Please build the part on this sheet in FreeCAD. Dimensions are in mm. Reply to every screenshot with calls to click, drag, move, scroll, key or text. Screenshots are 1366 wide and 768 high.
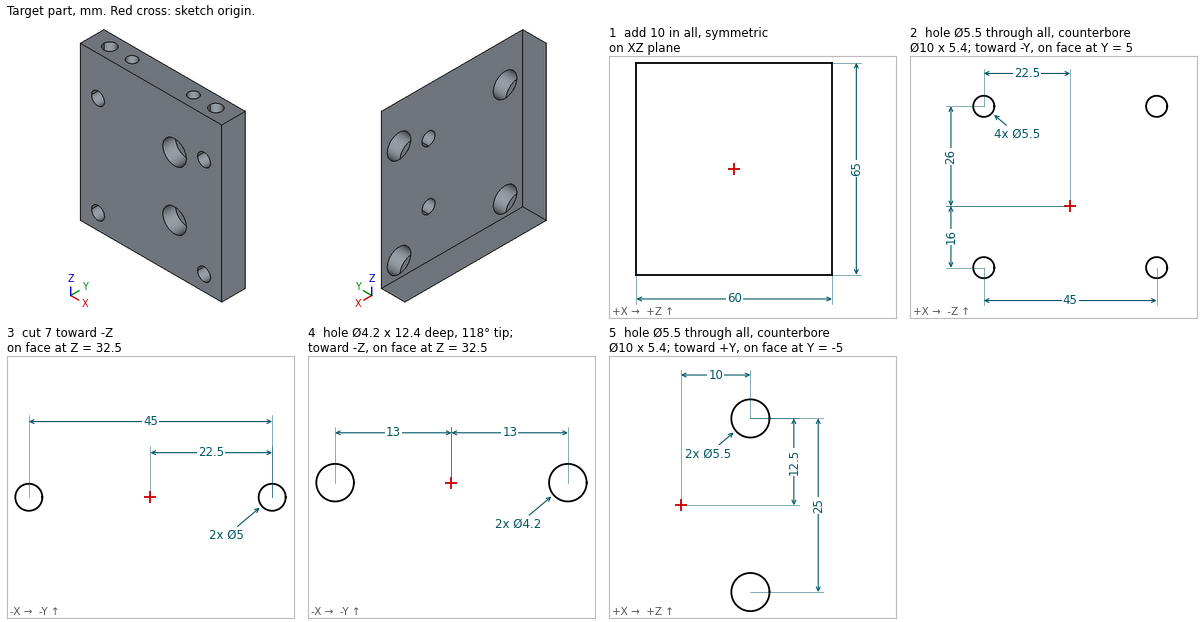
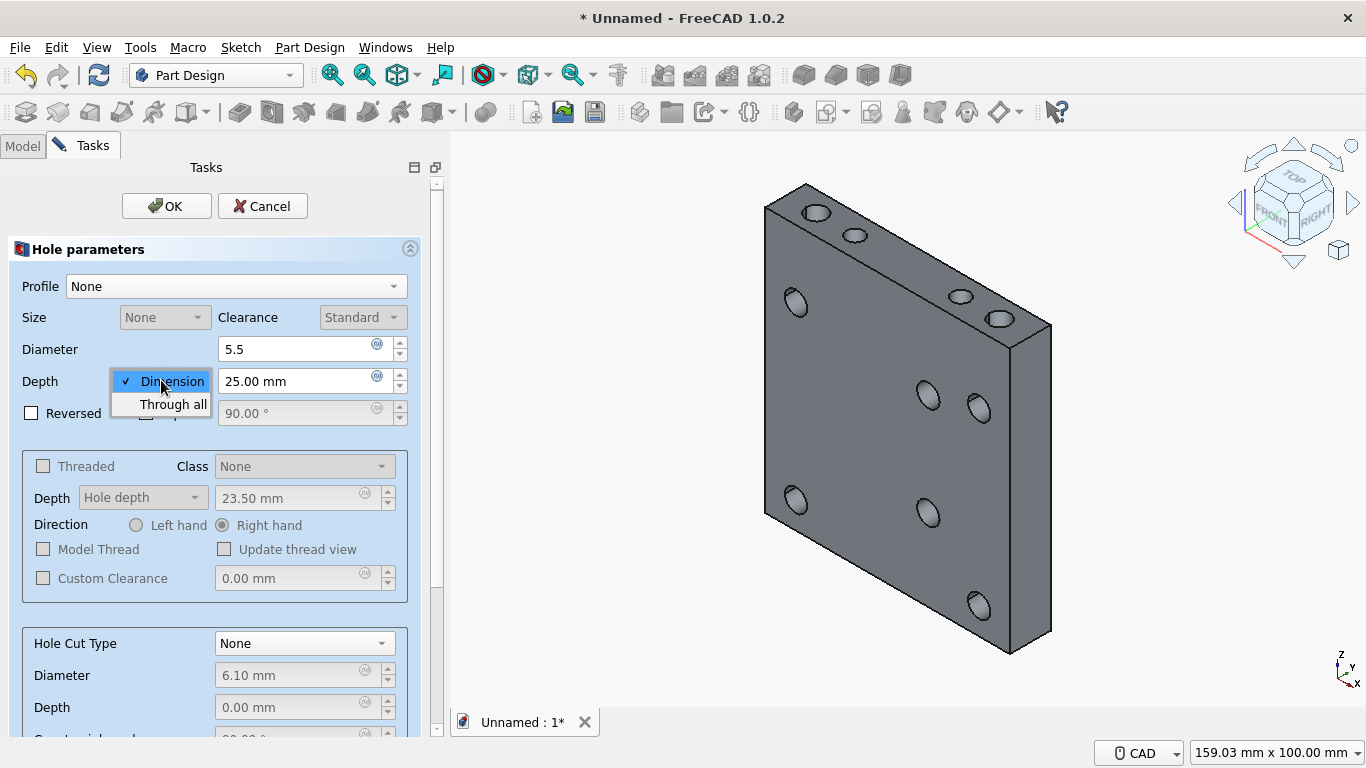
click(160, 404)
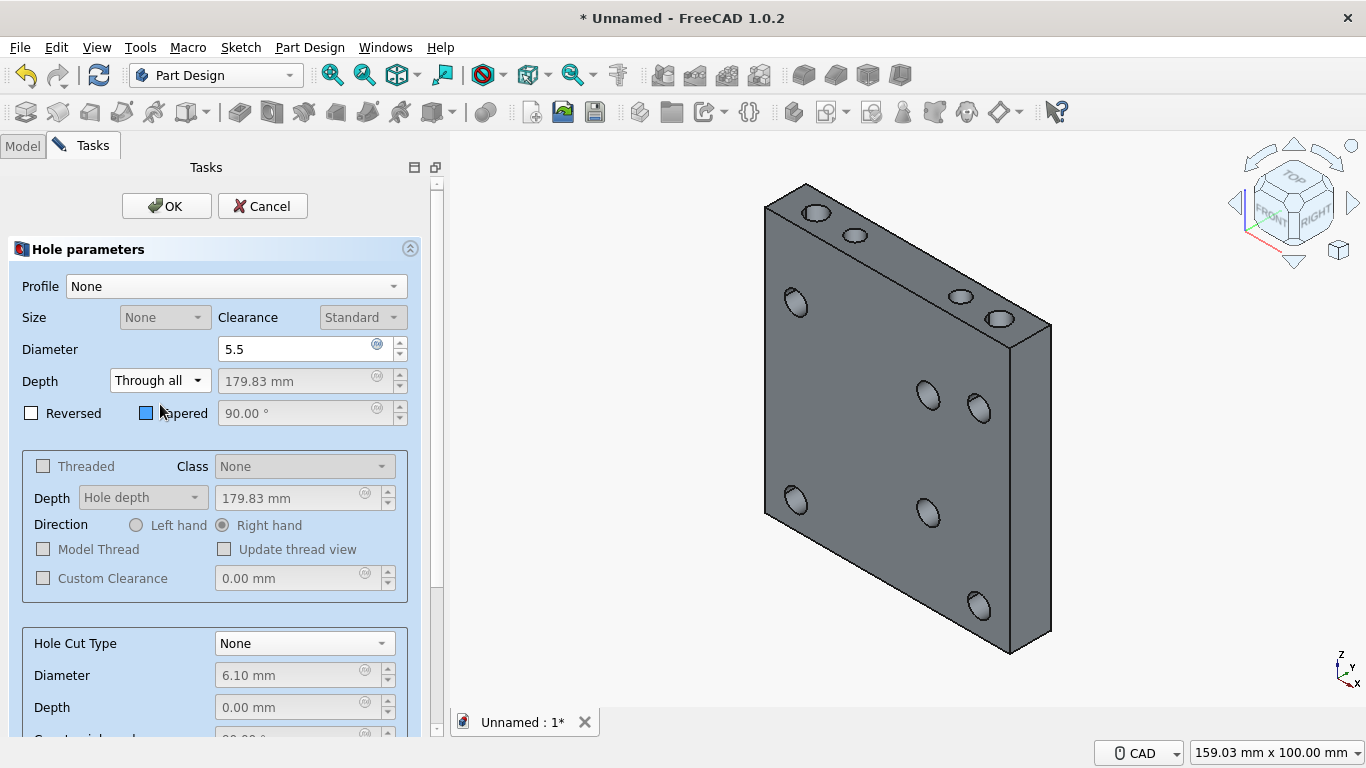
click(306, 644)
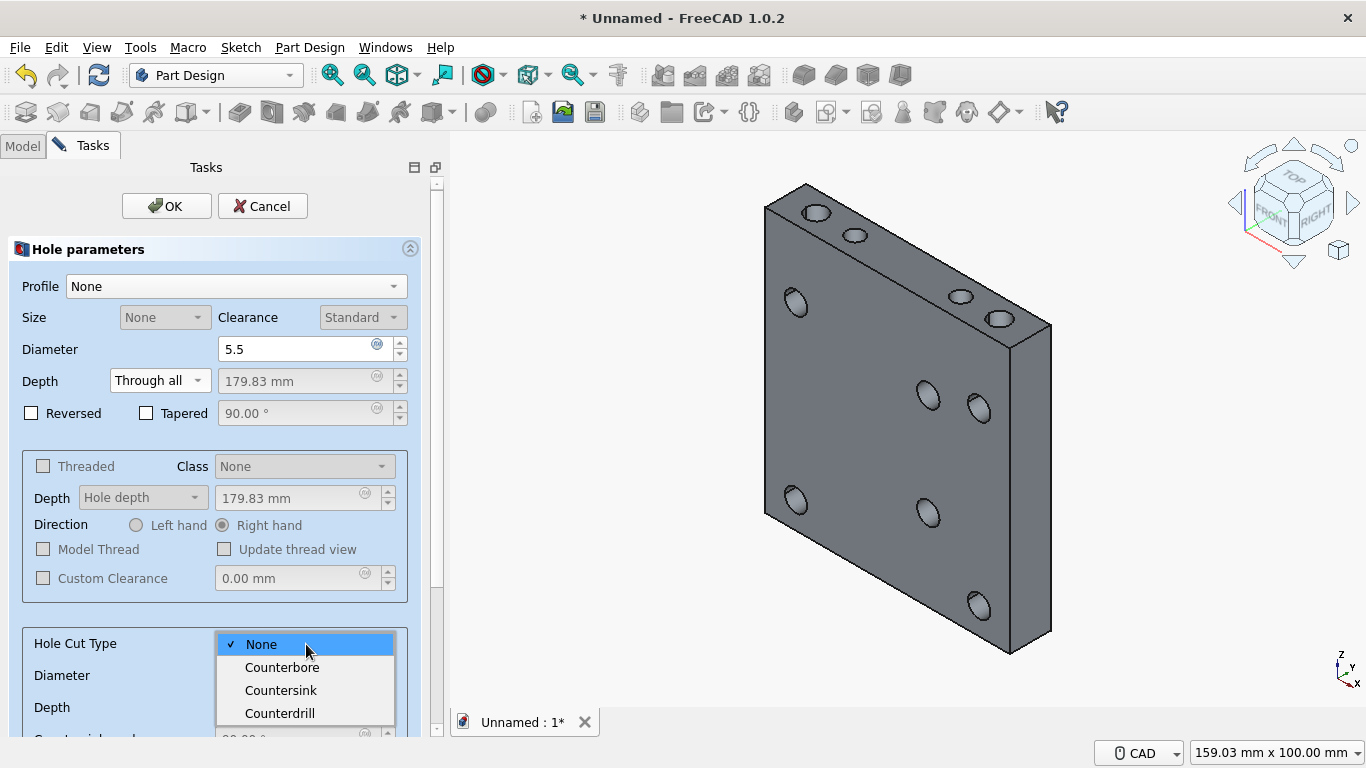
click(304, 668)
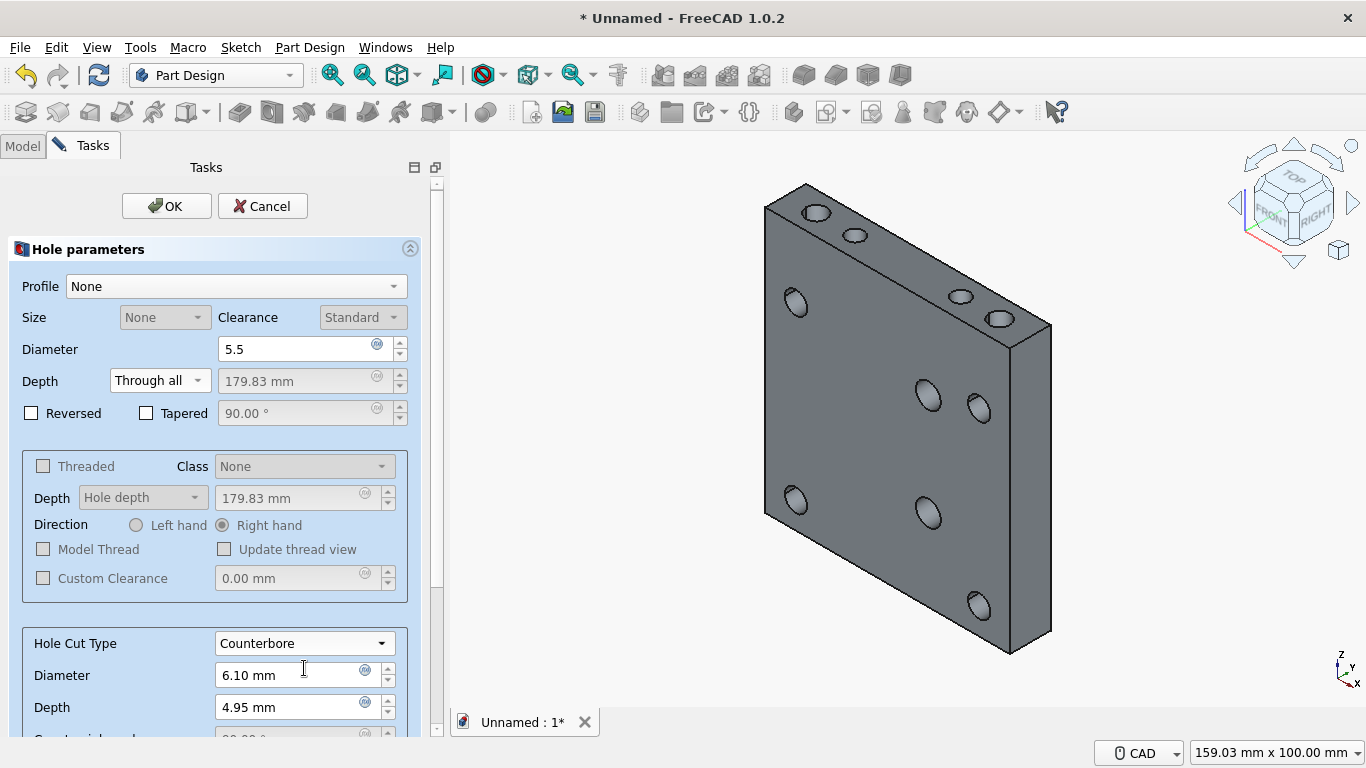
triple_click(298, 675)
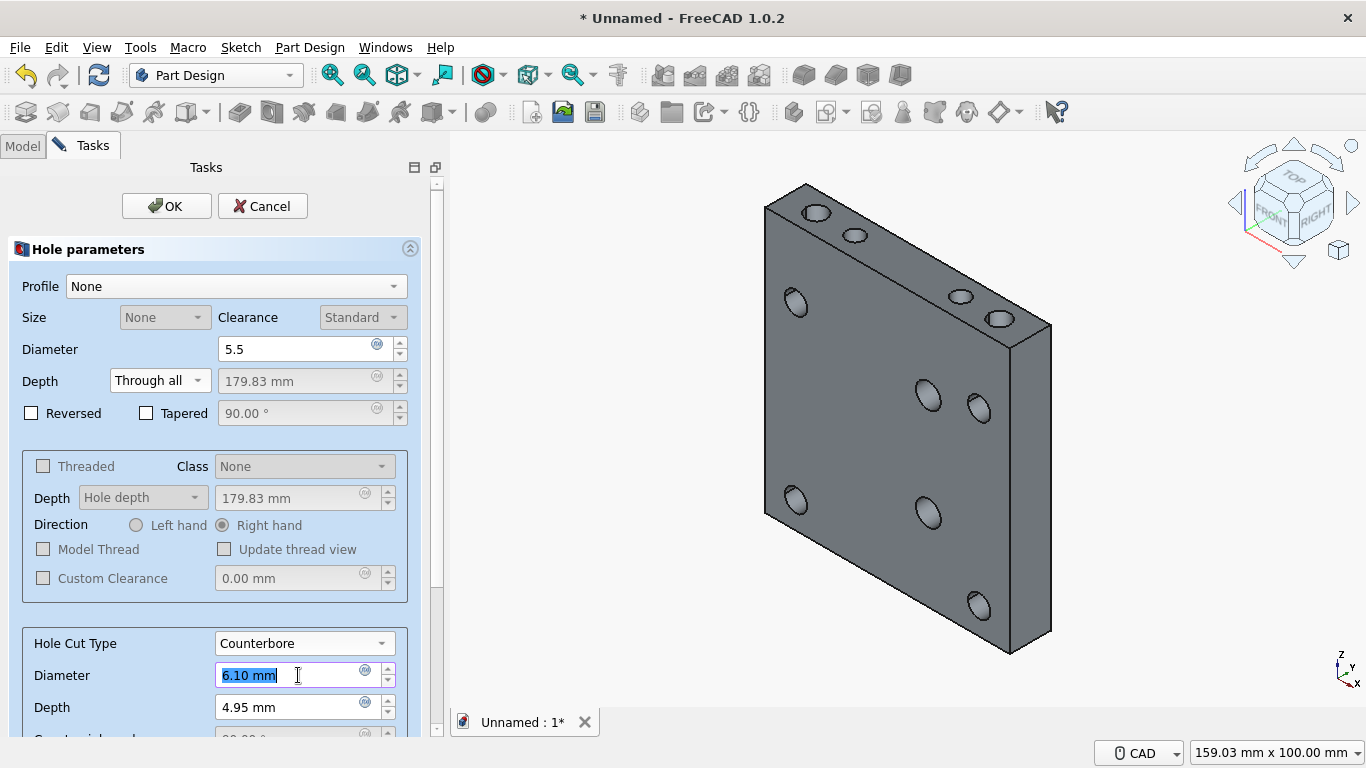
text(10)
key(Tab)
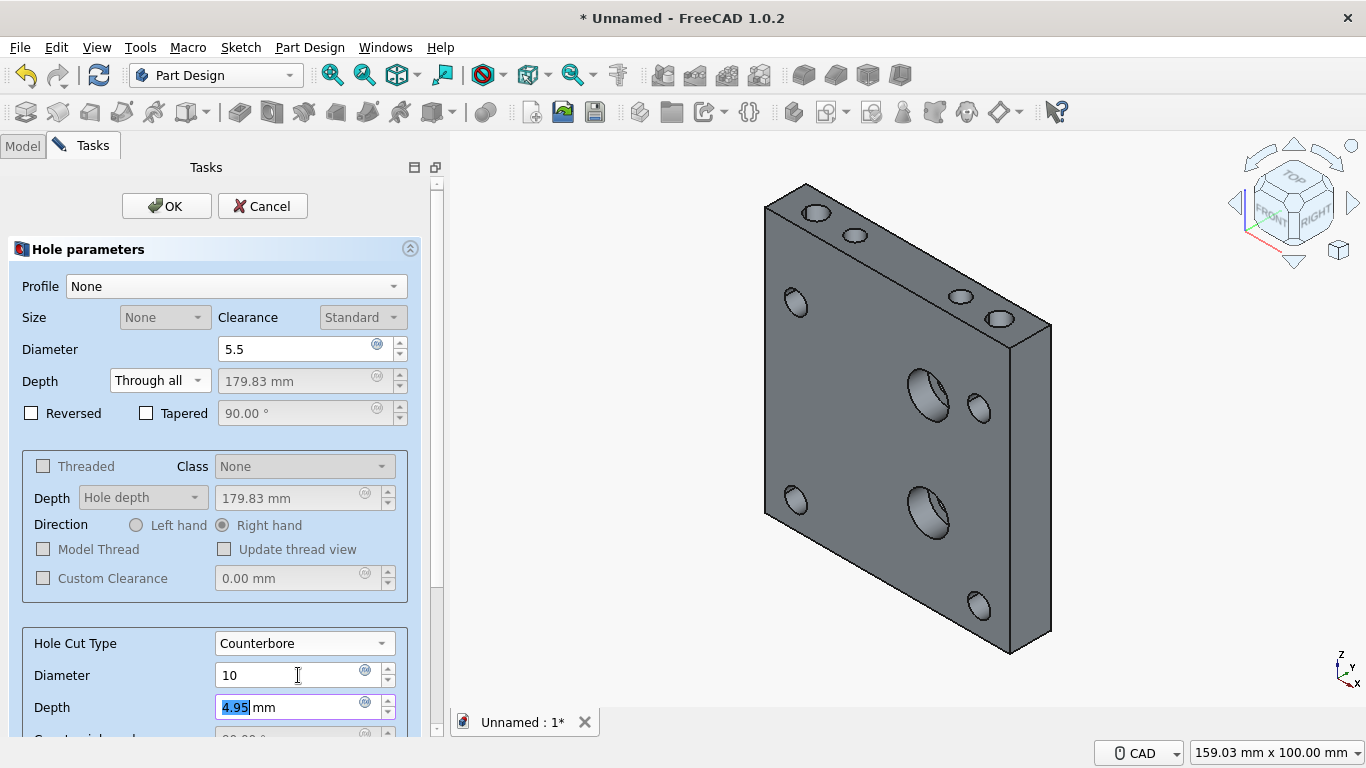
text(5.4)
key(Tab)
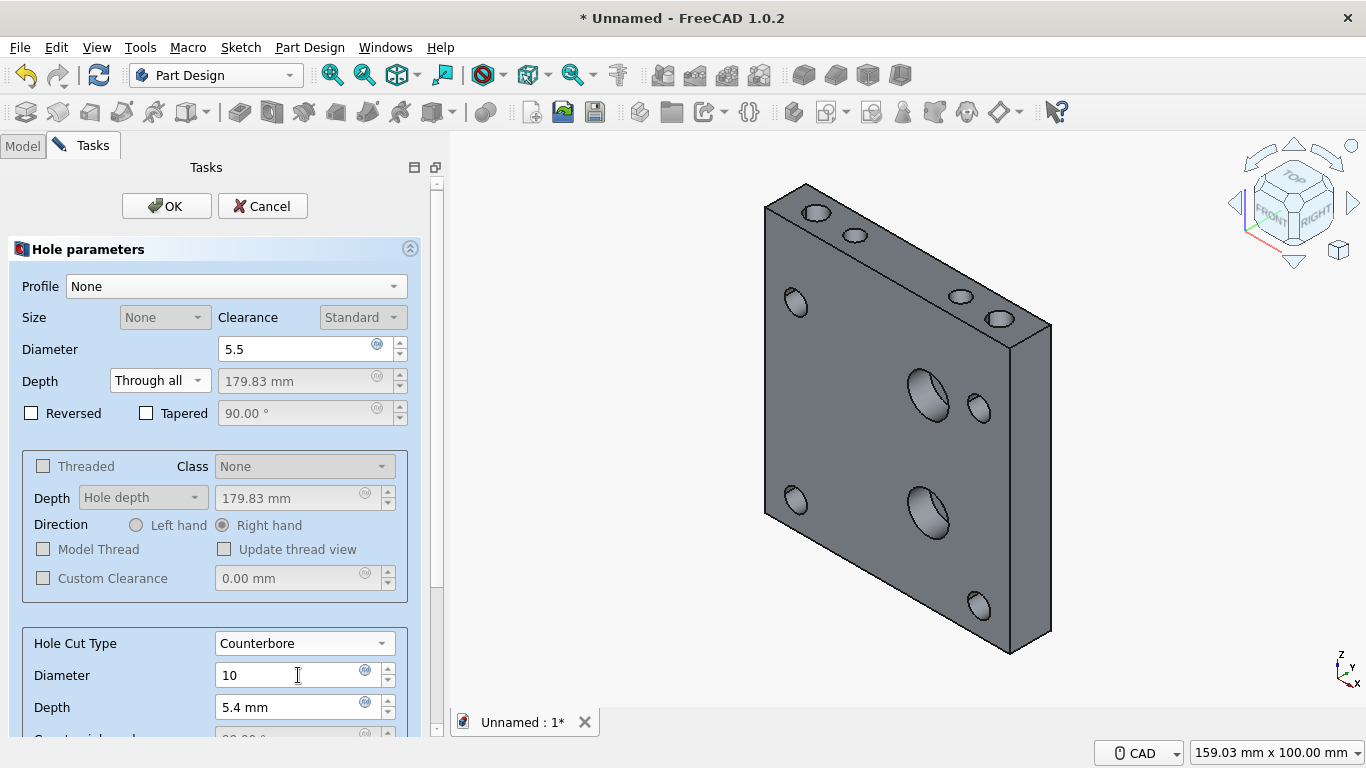
click(167, 206)